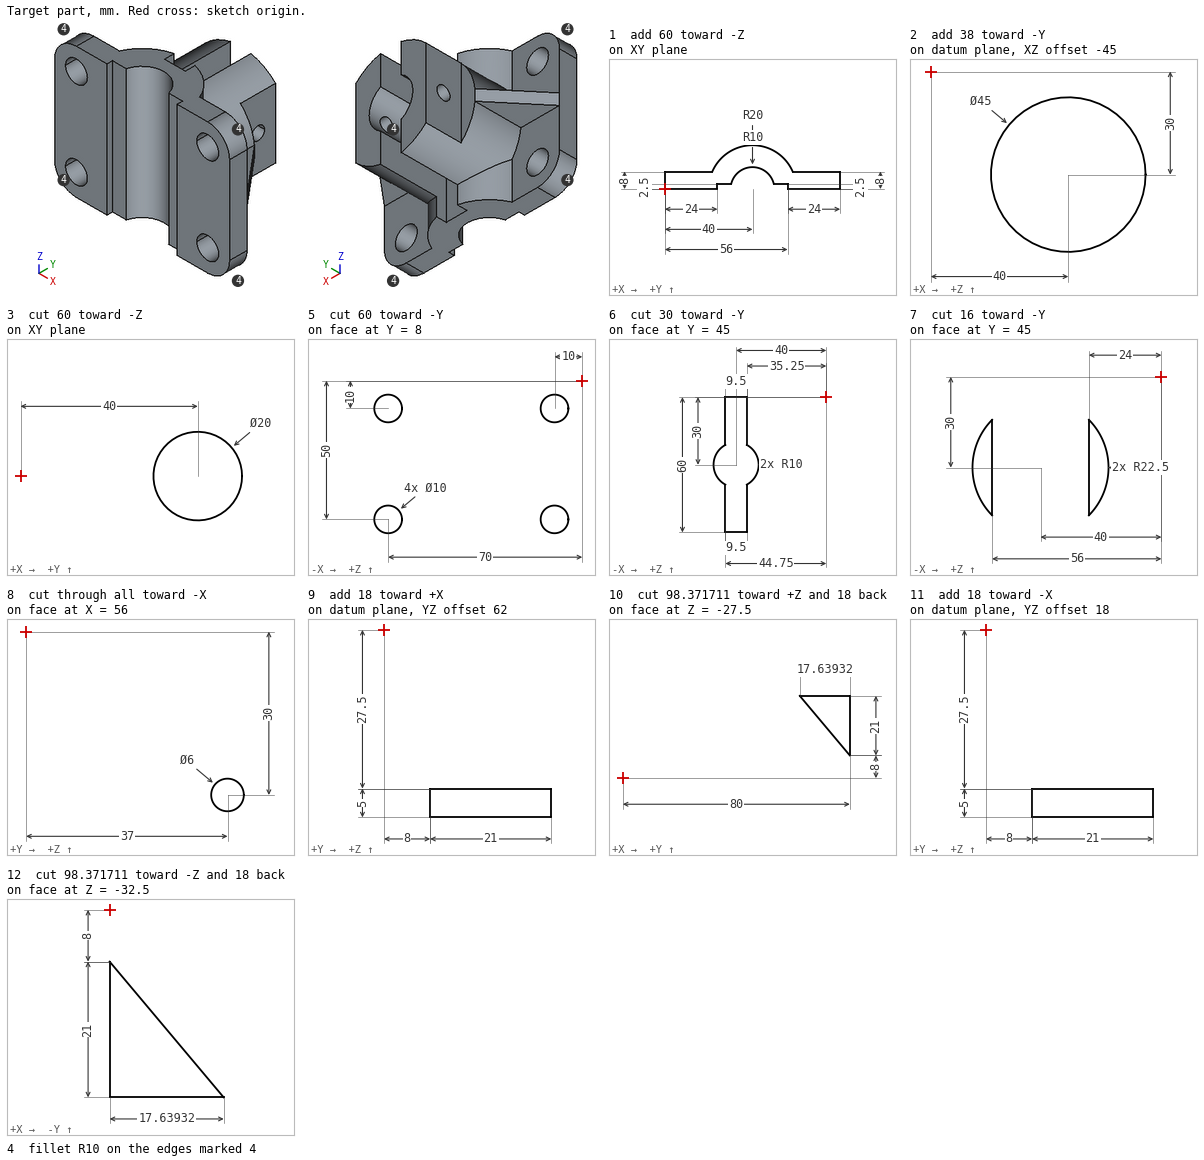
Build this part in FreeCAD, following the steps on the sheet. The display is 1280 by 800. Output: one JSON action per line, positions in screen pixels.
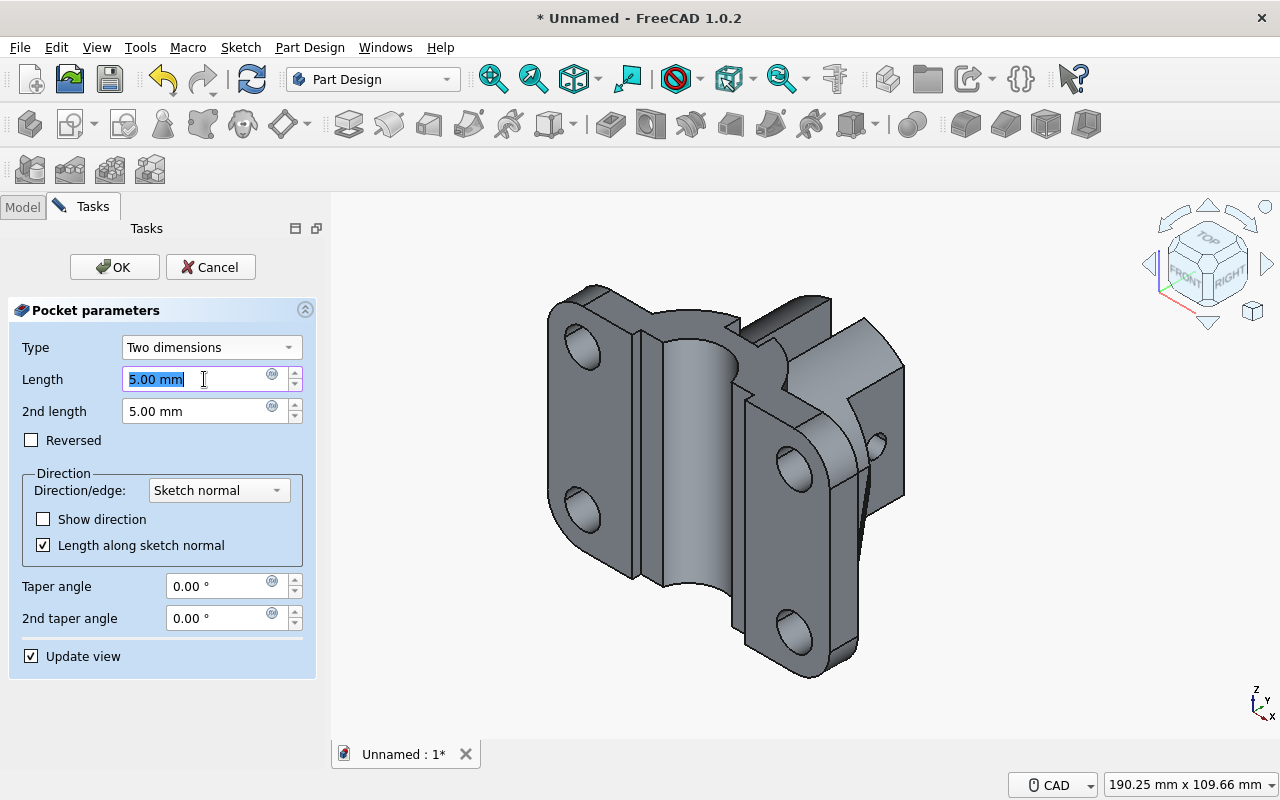
{"action": "type", "text": "98.371711"}
{"action": "key", "text": "Tab"}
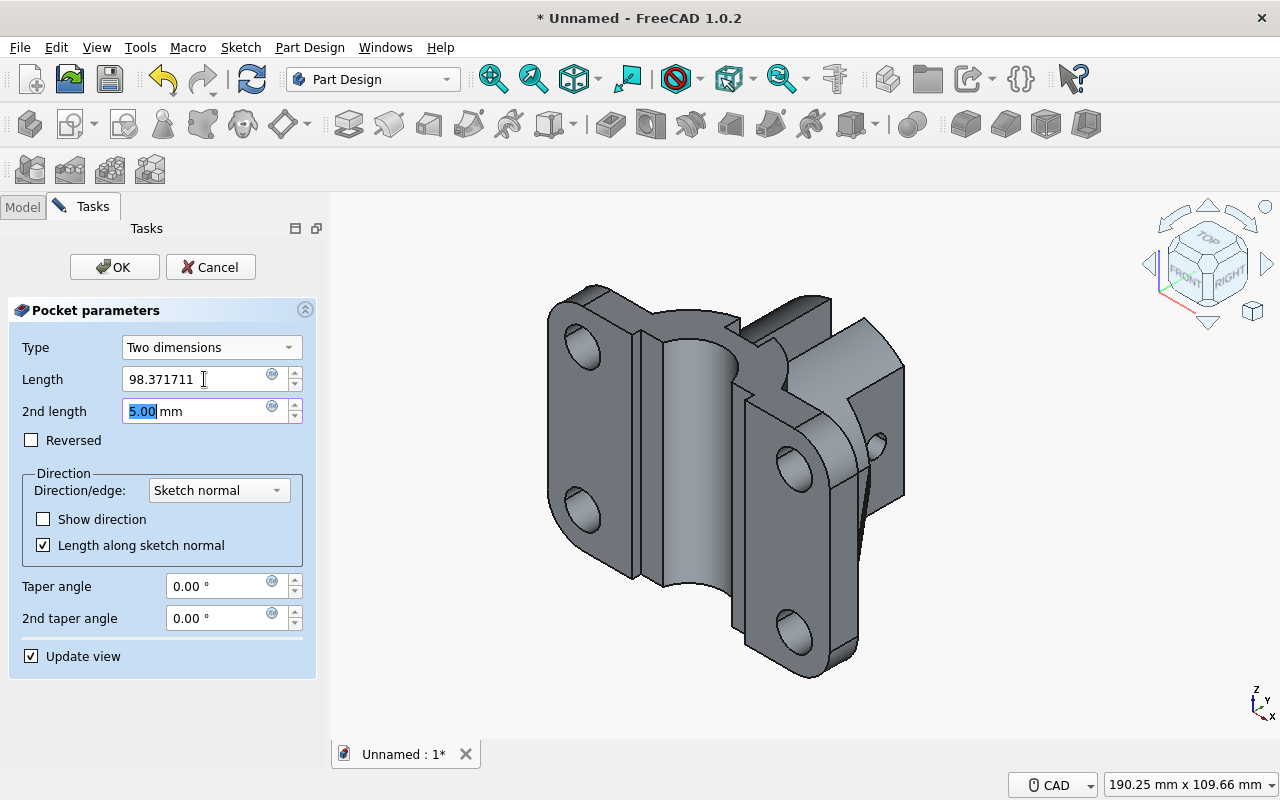
{"action": "type", "text": "18"}
{"action": "key", "text": "Tab"}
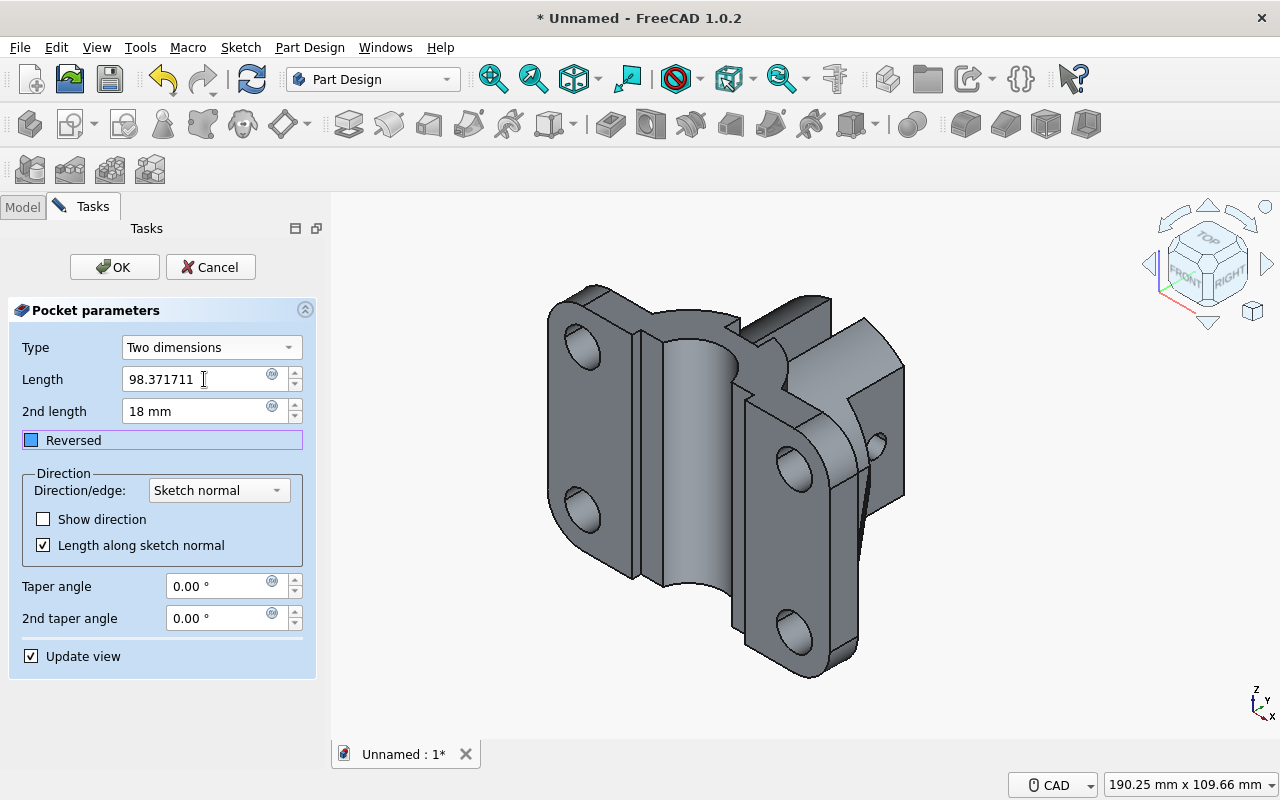
{"action": "left_click", "coordinate": [30, 440]}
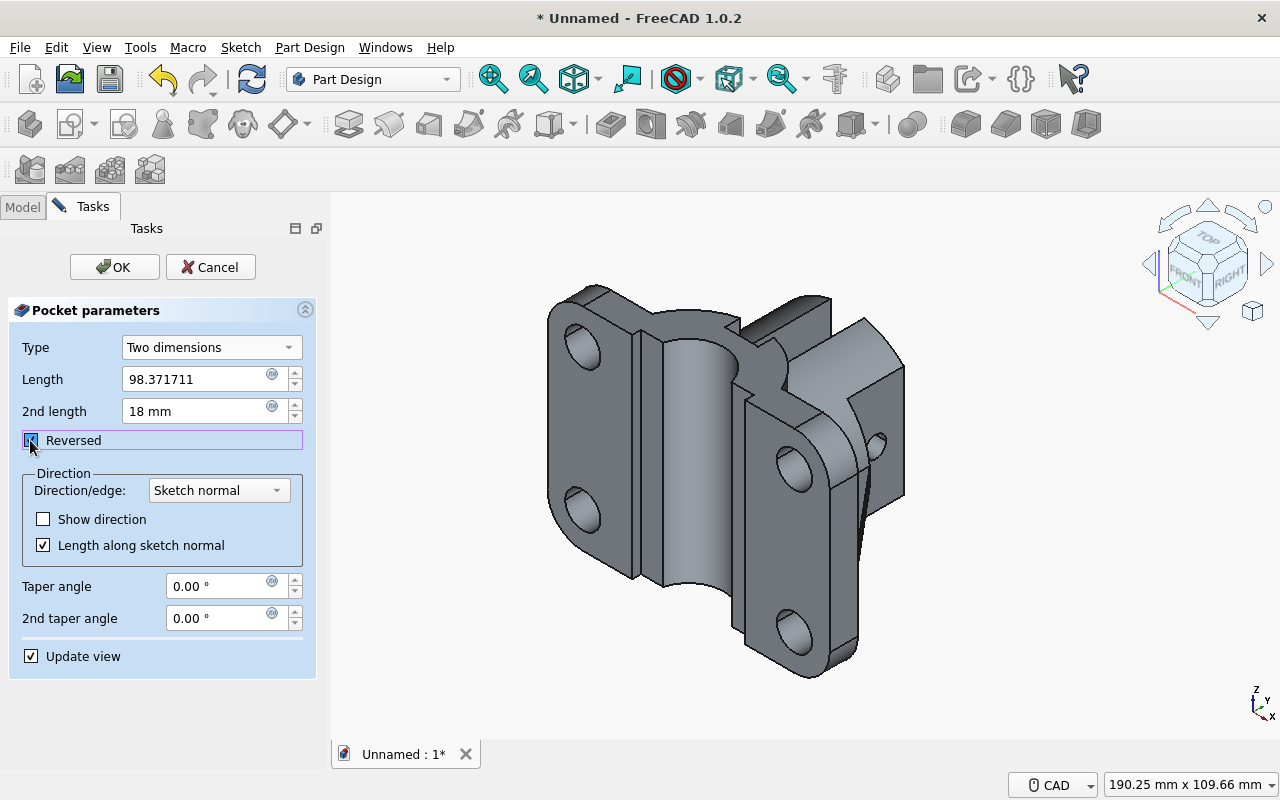
{"action": "left_click", "coordinate": [115, 267]}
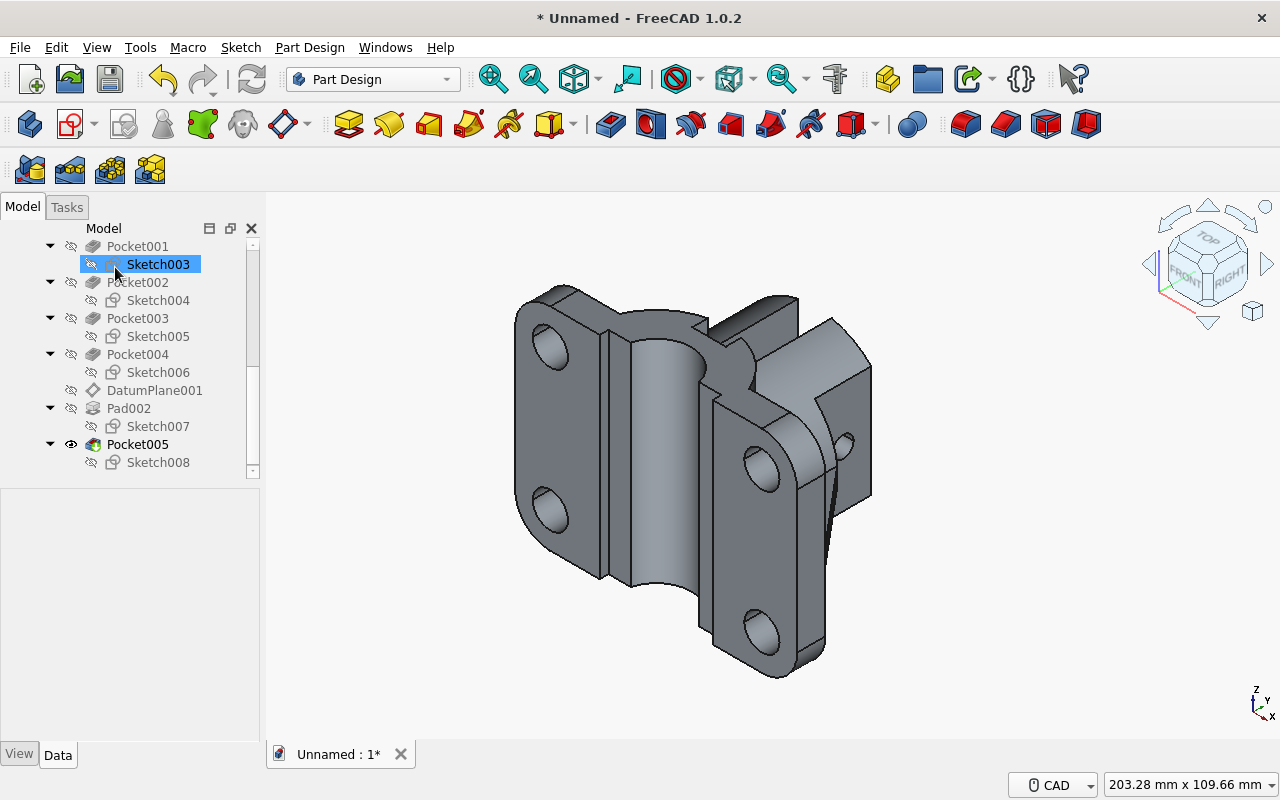
{"action": "scroll", "coordinate": [140, 350], "scroll_direction": "down", "scroll_amount": 3}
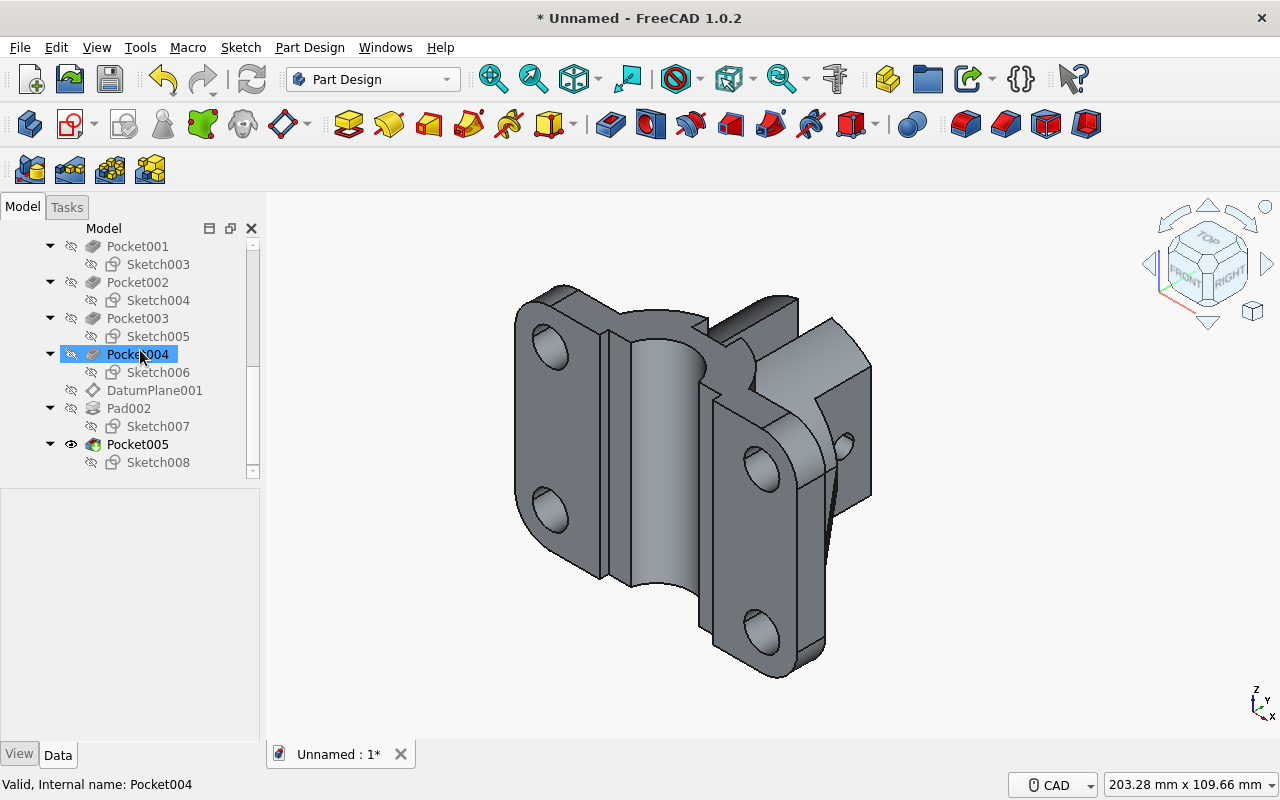
{"action": "scroll", "coordinate": [140, 350], "scroll_direction": "up", "scroll_amount": 15}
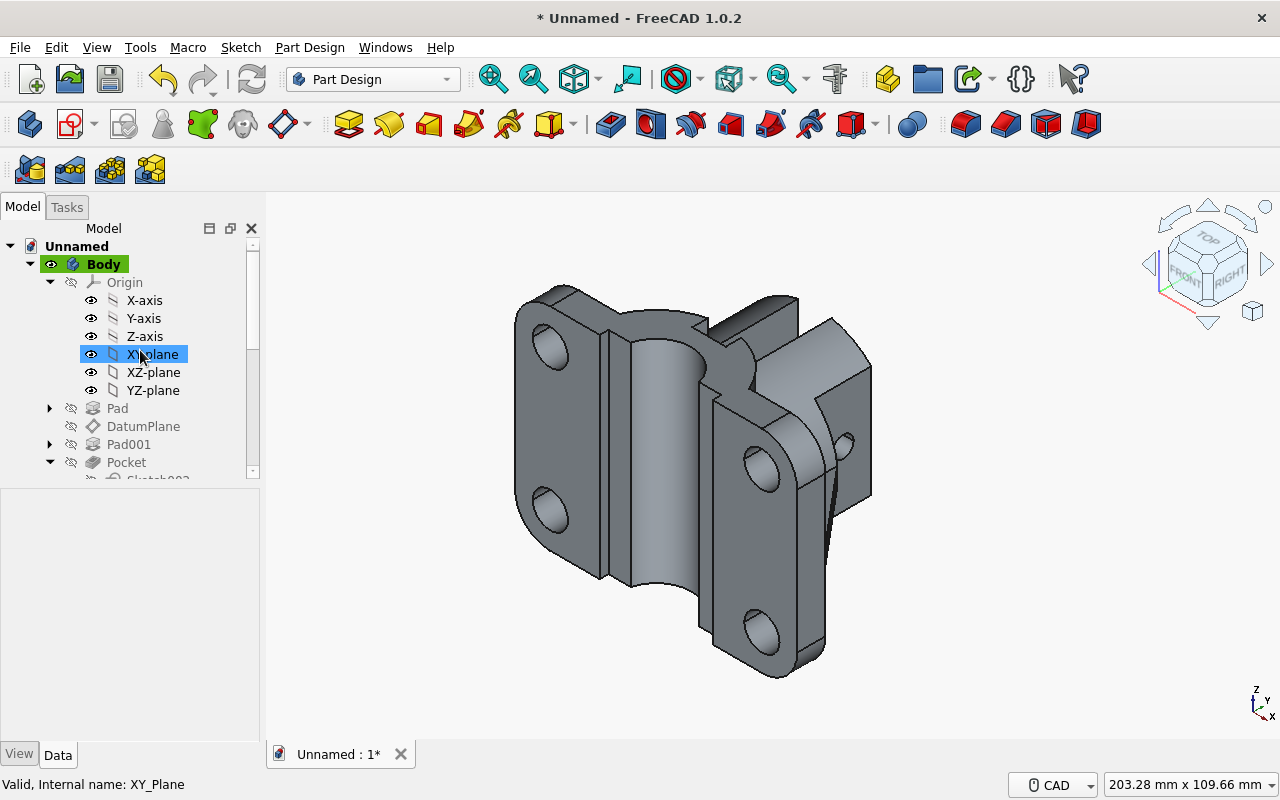
{"action": "left_click", "coordinate": [136, 390]}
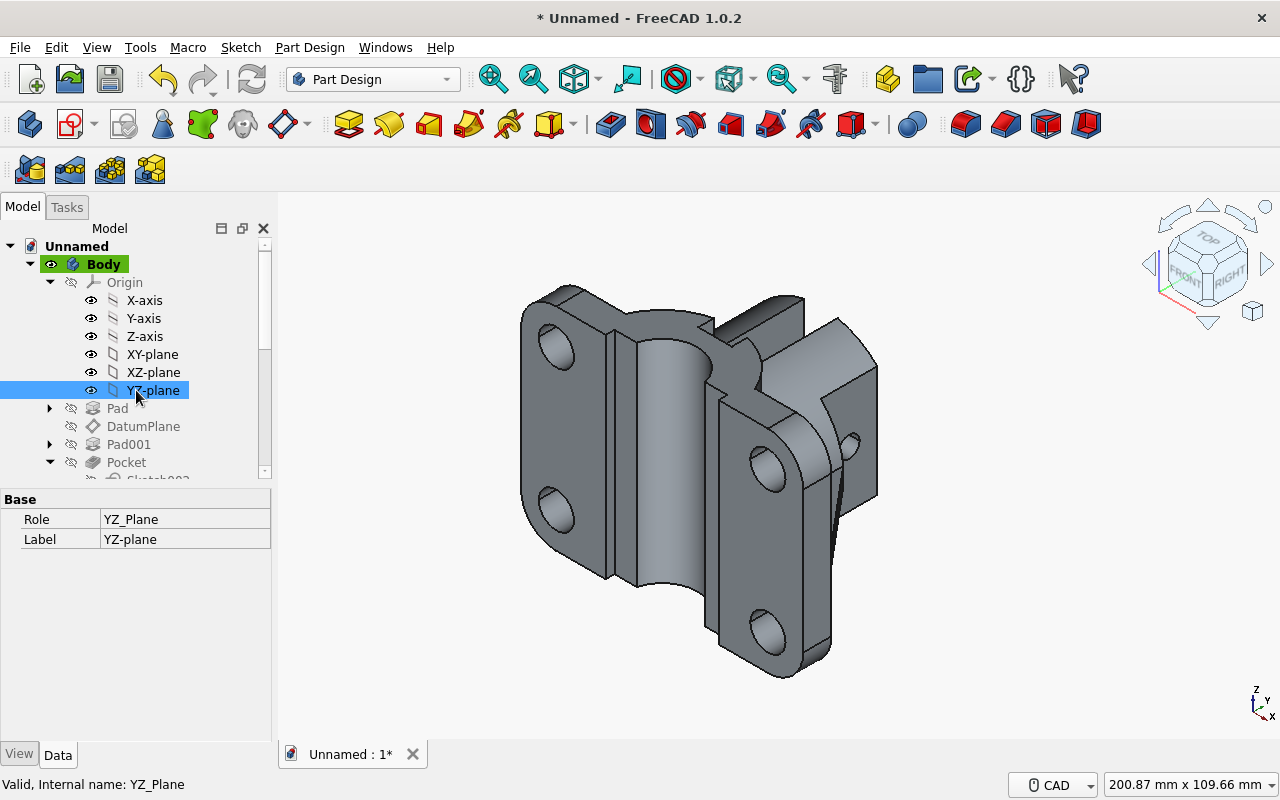
{"action": "left_click", "coordinate": [284, 124]}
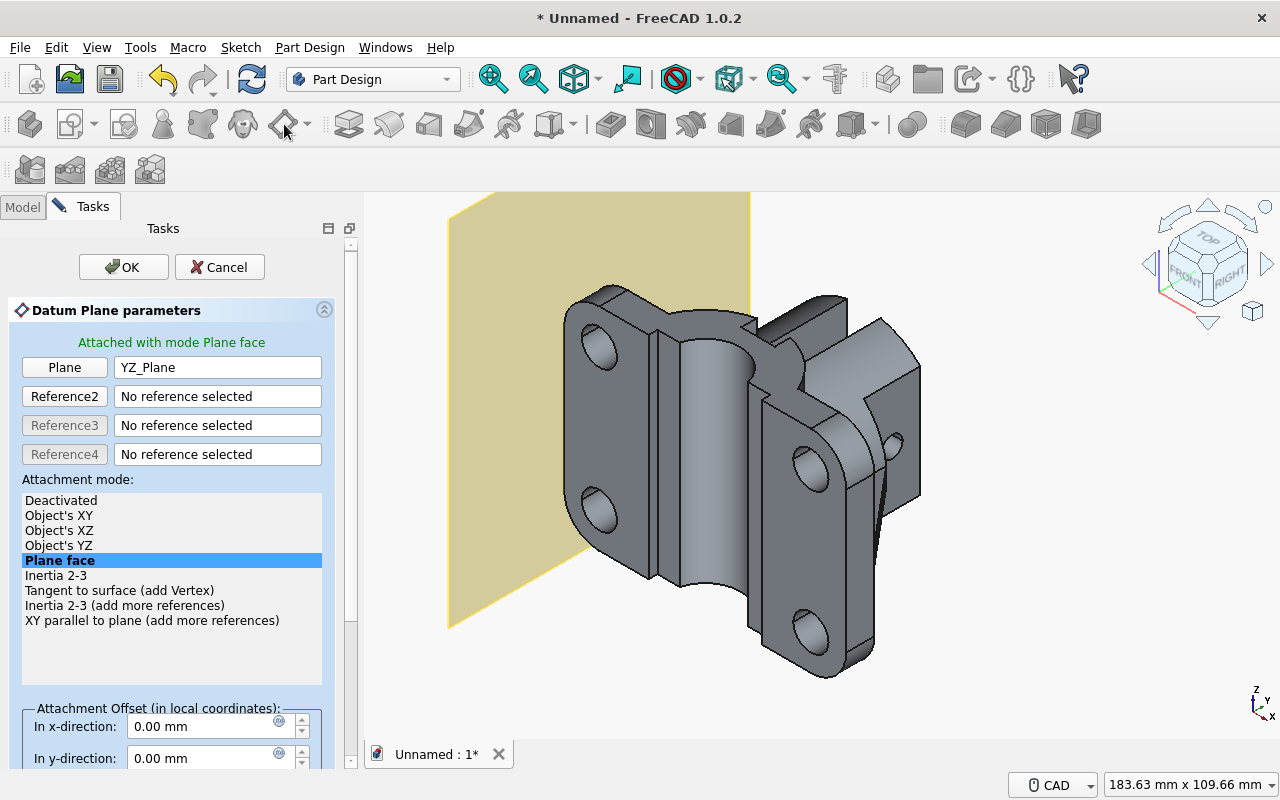
{"action": "scroll", "coordinate": [351, 503], "scroll_direction": "down", "scroll_amount": 2}